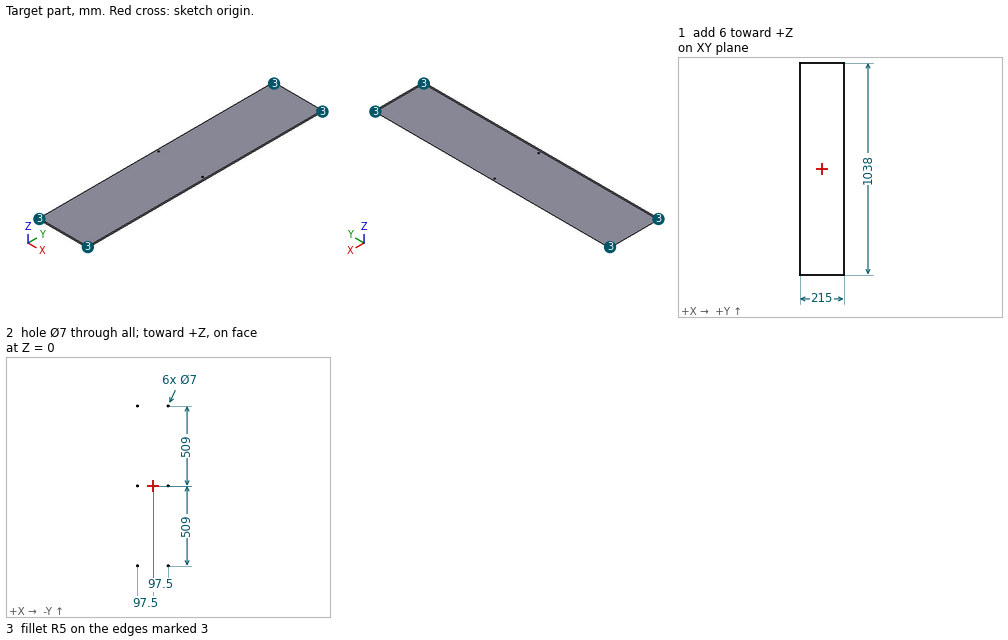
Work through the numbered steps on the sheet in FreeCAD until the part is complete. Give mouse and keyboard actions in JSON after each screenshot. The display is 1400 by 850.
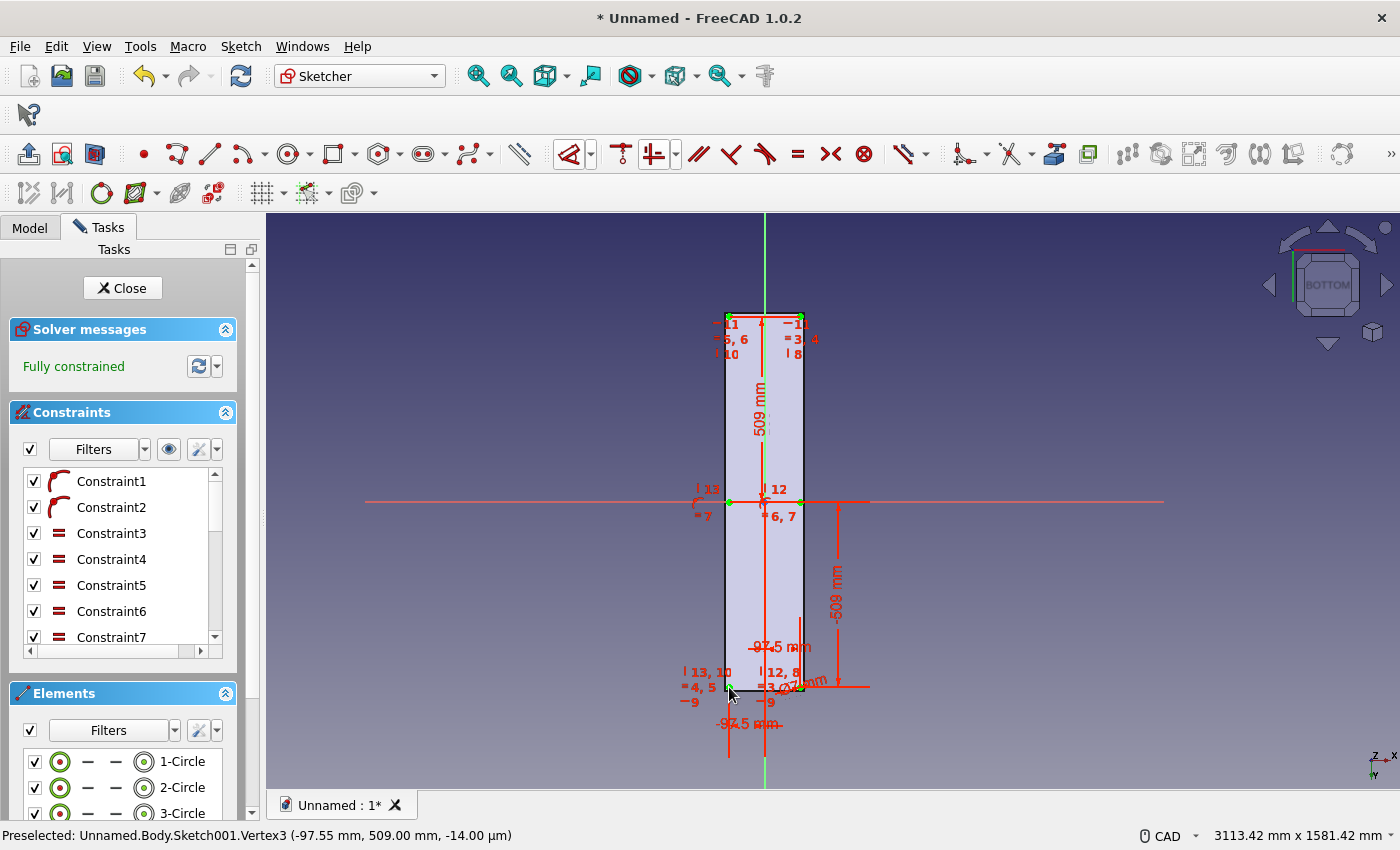
{"action": "left_click", "coordinate": [123, 288]}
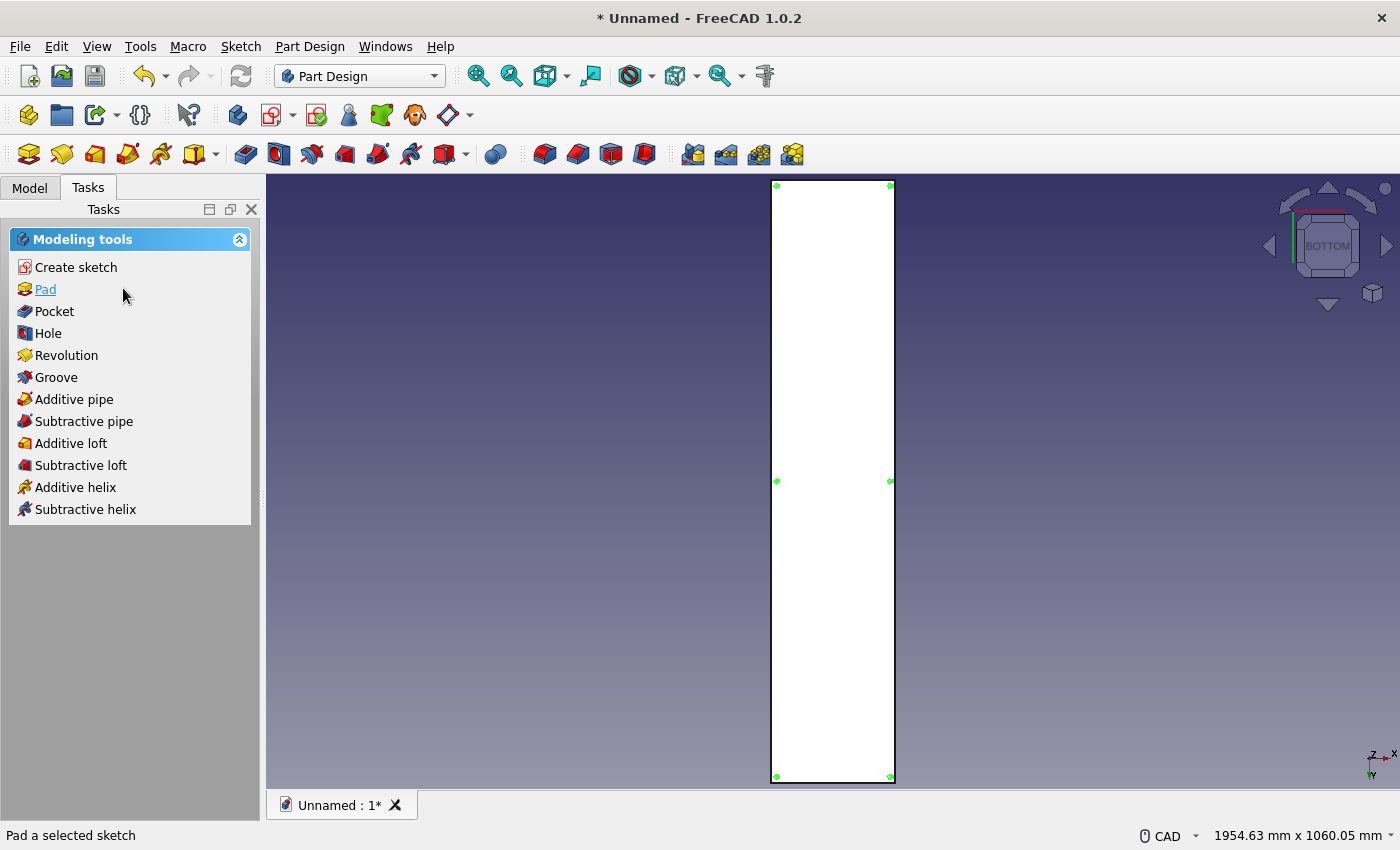
{"action": "left_click", "coordinate": [279, 154]}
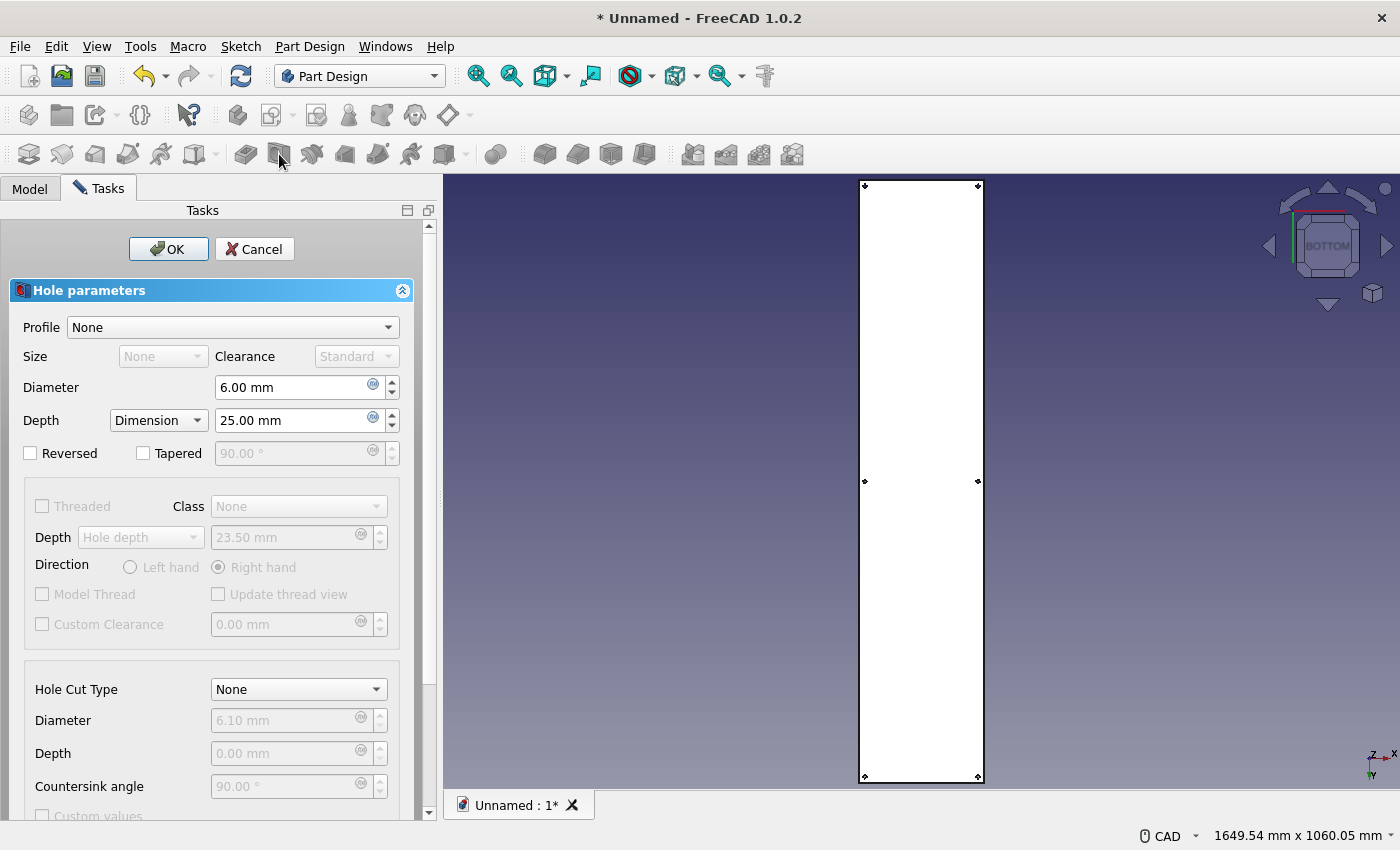
{"action": "triple_click", "coordinate": [300, 388]}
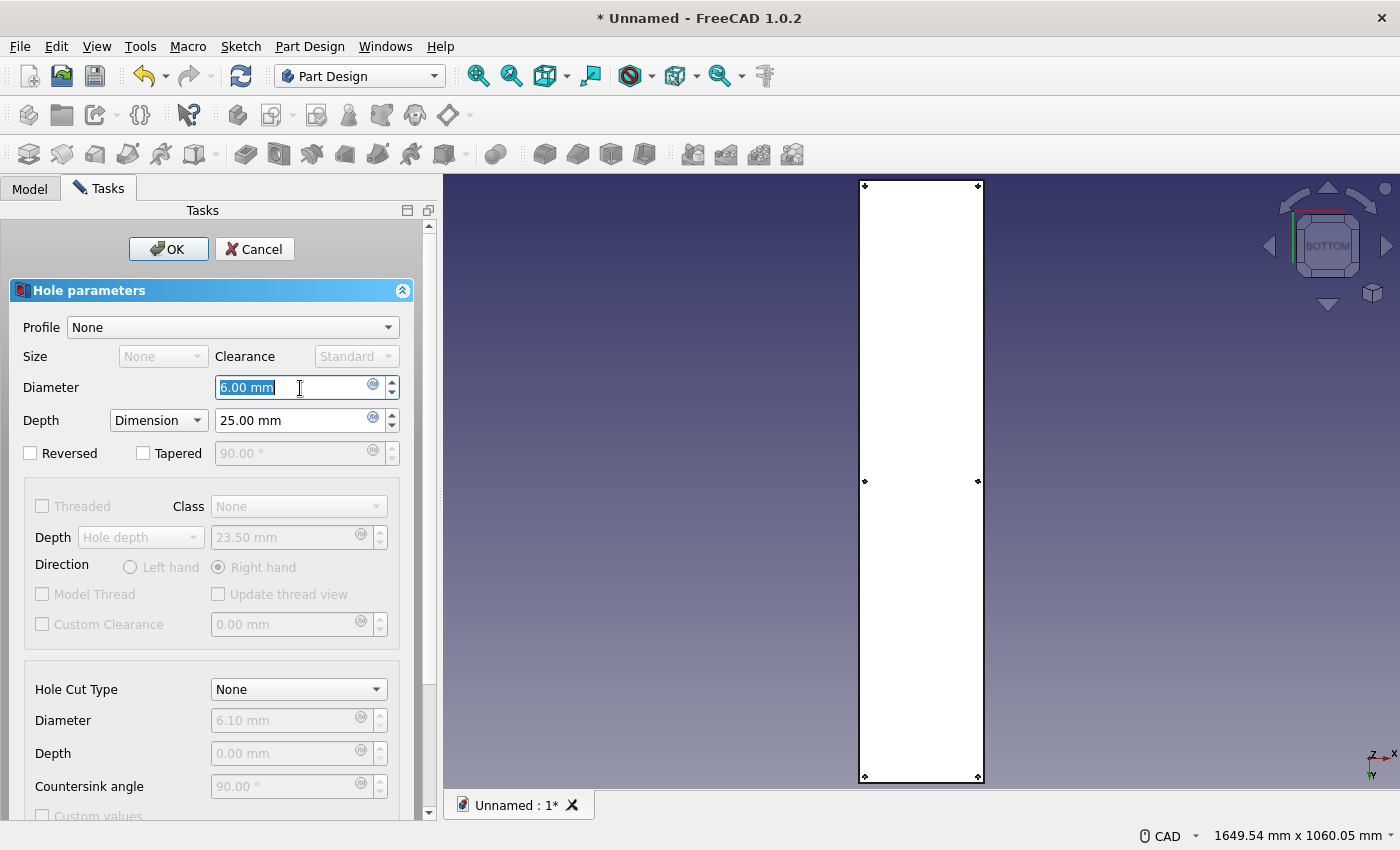
{"action": "type", "text": "7"}
{"action": "key", "text": "Tab"}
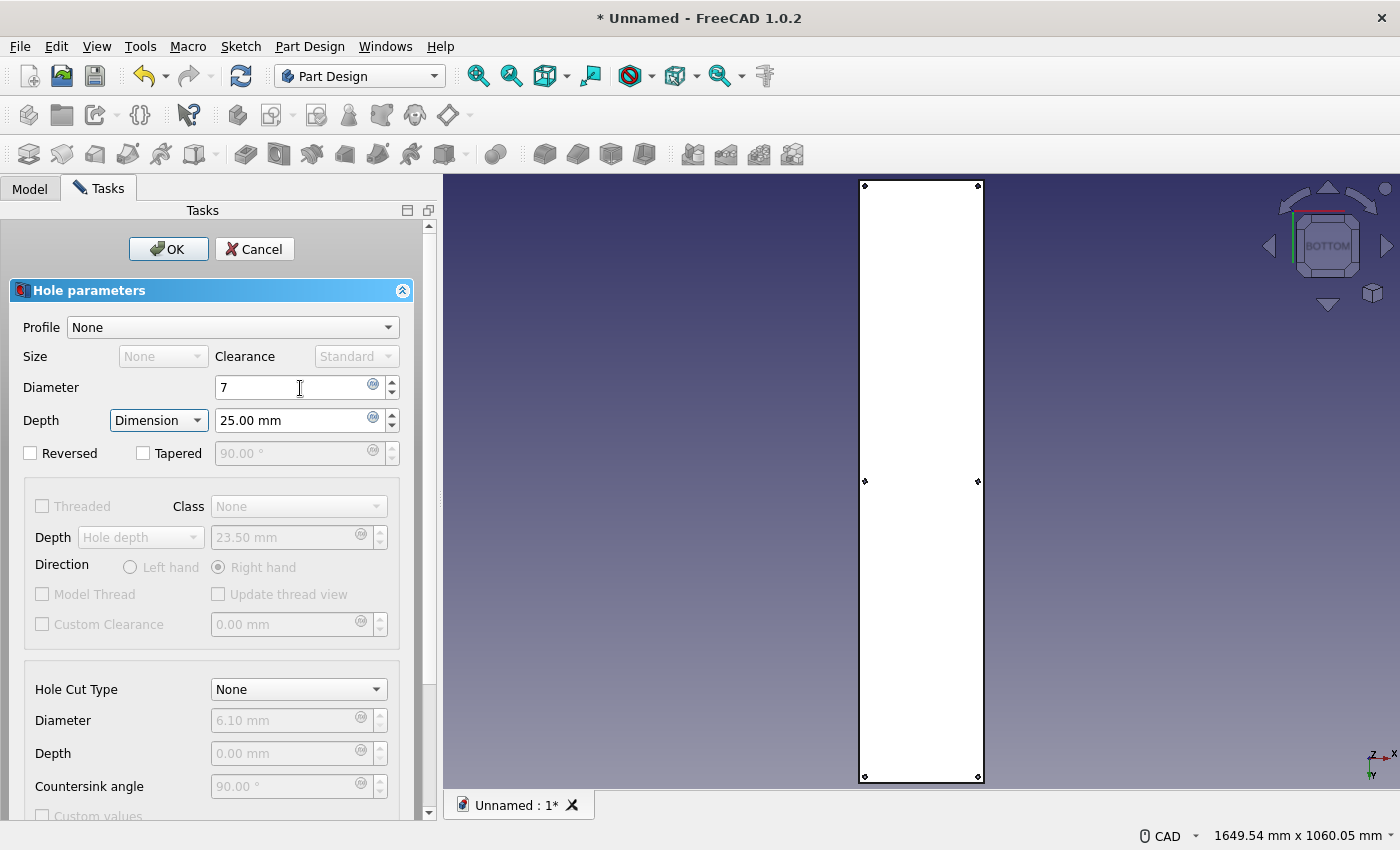
{"action": "left_click", "coordinate": [160, 420]}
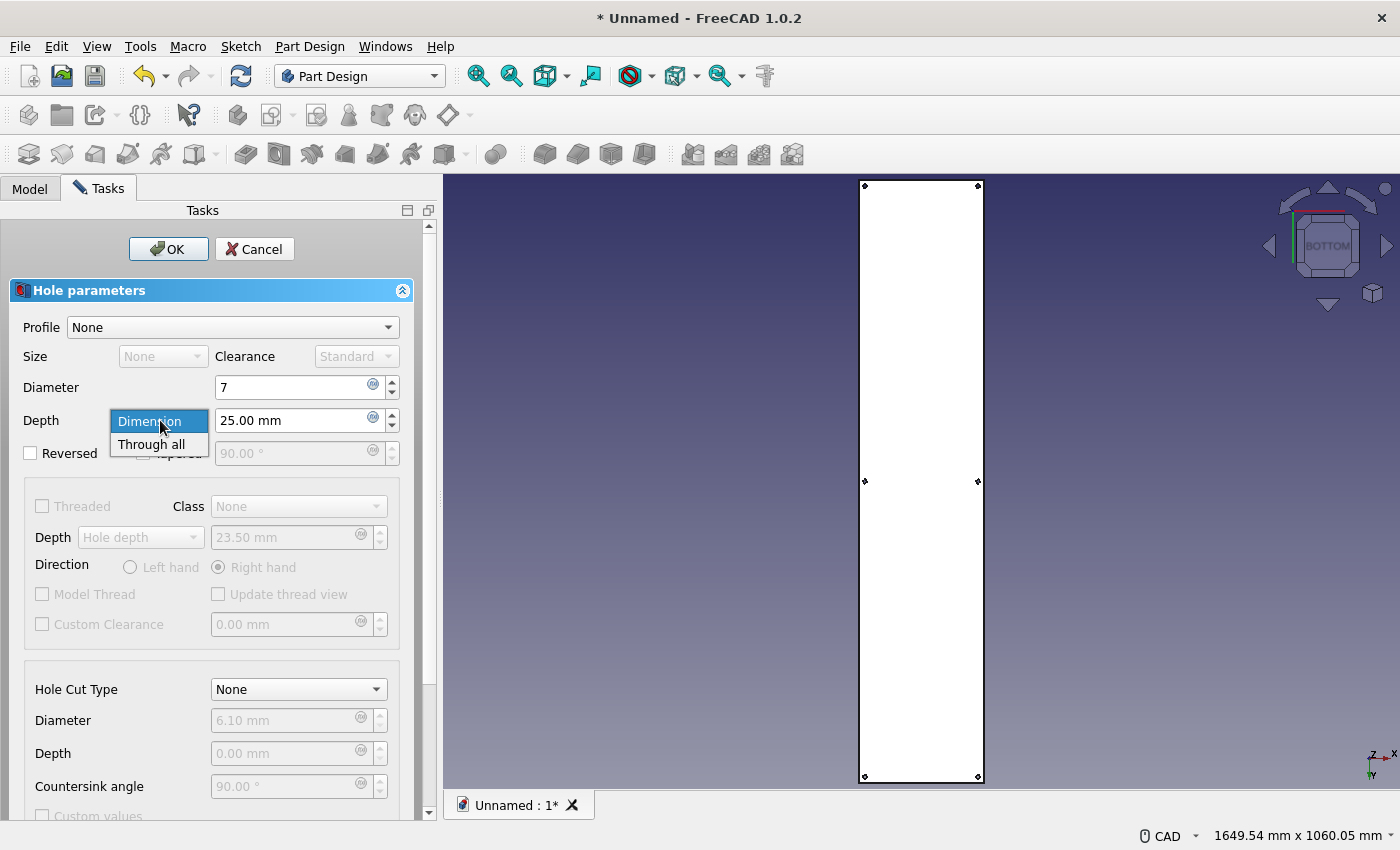
{"action": "left_click", "coordinate": [158, 444]}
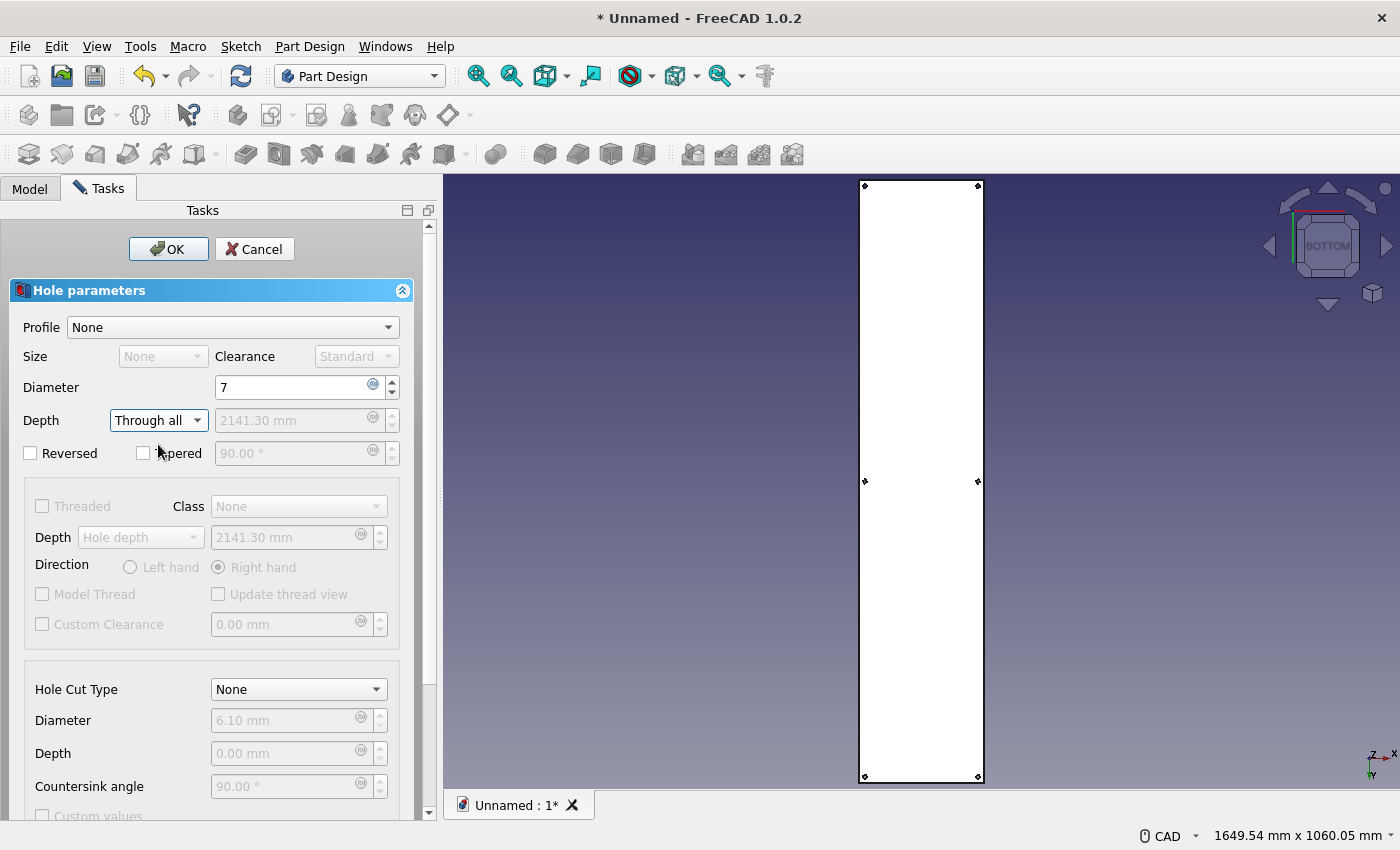
{"action": "left_click", "coordinate": [169, 249]}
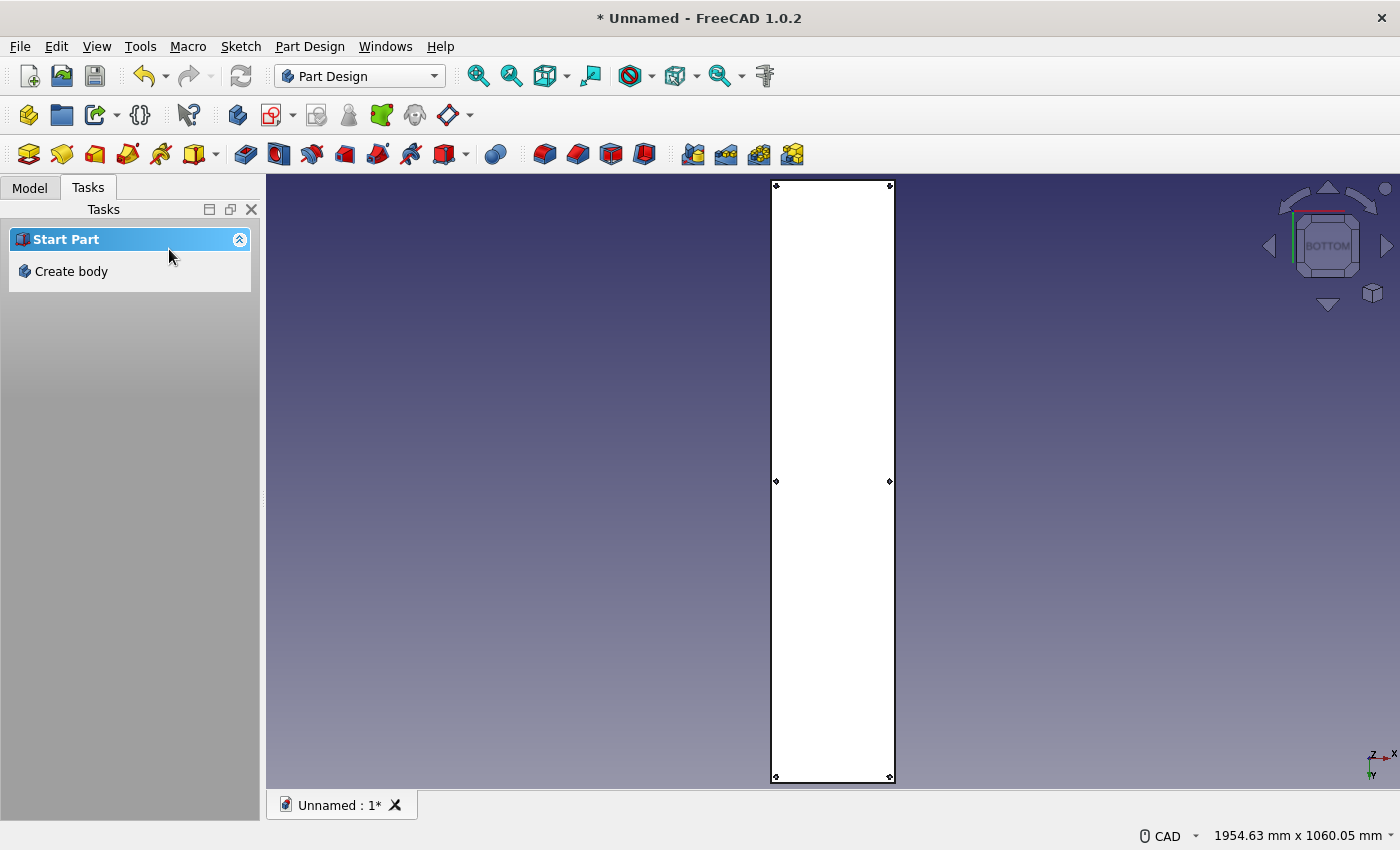
{"action": "key", "text": "0"}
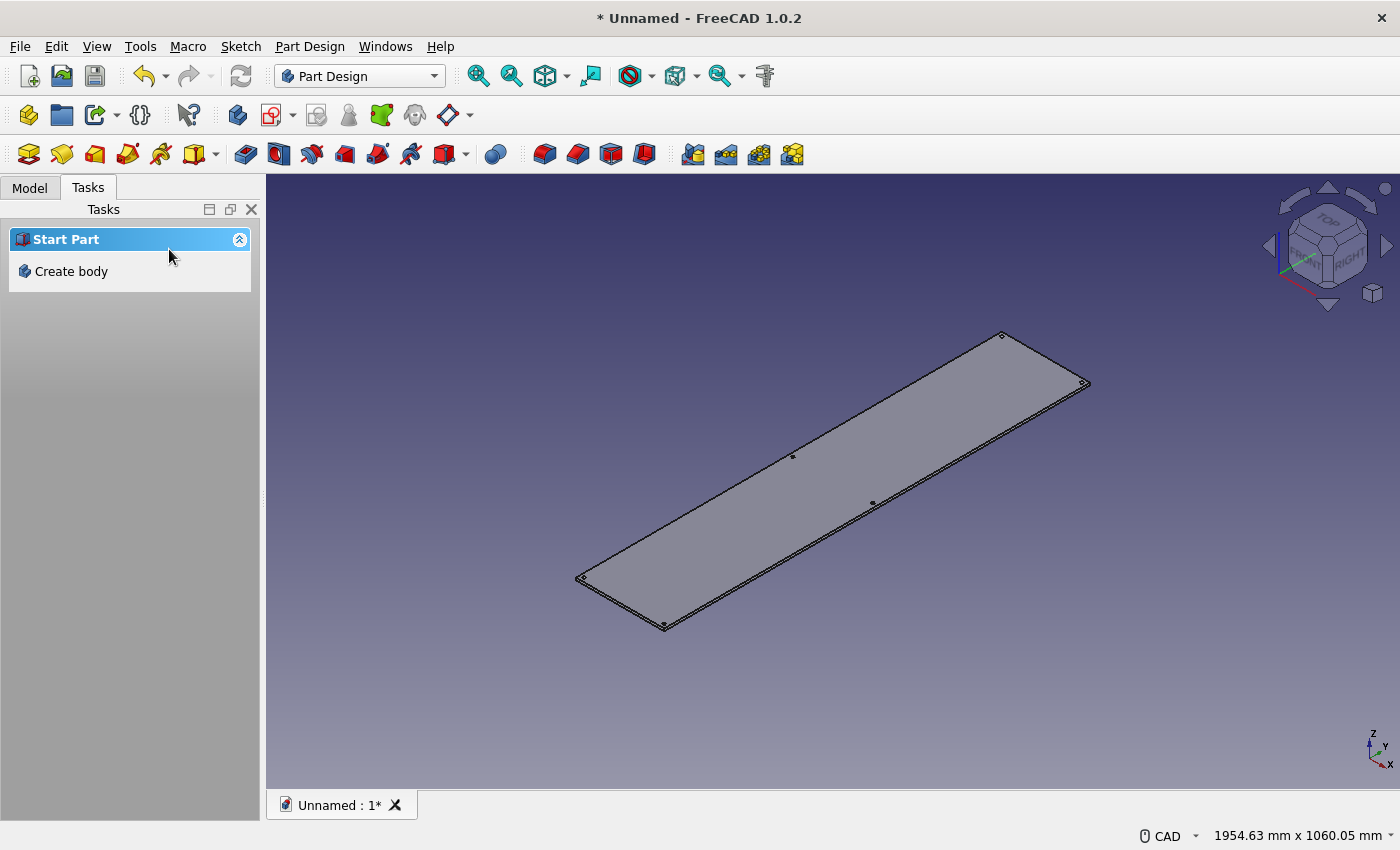
{"action": "scroll", "coordinate": [664, 629], "scroll_direction": "up", "scroll_amount": 13}